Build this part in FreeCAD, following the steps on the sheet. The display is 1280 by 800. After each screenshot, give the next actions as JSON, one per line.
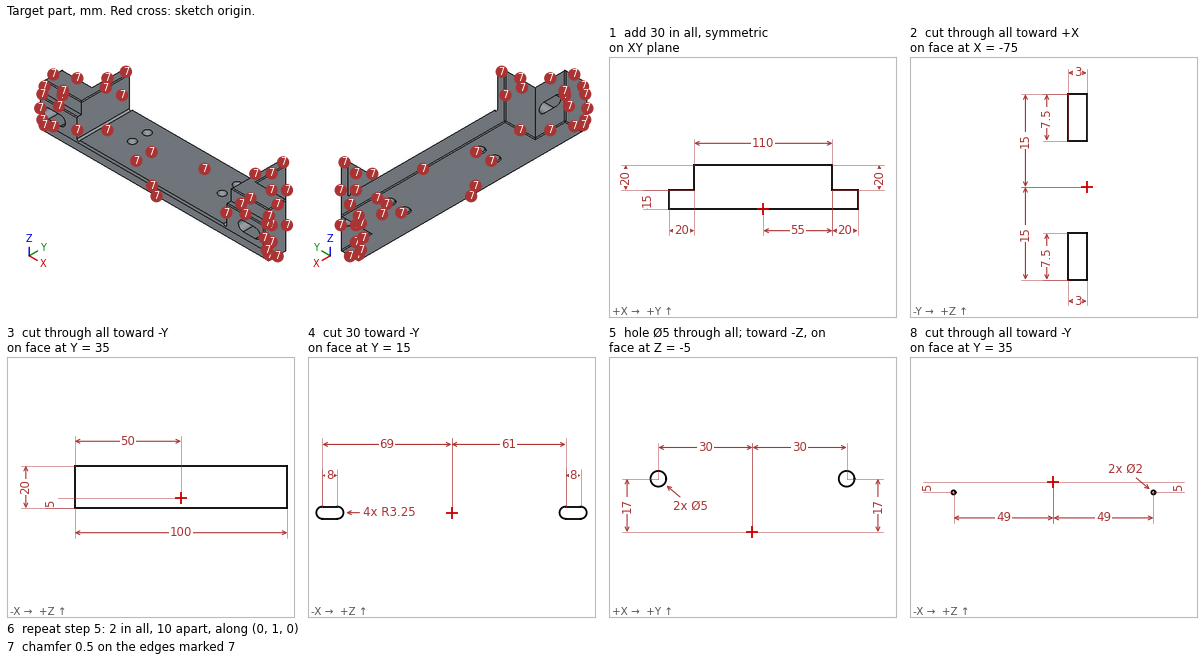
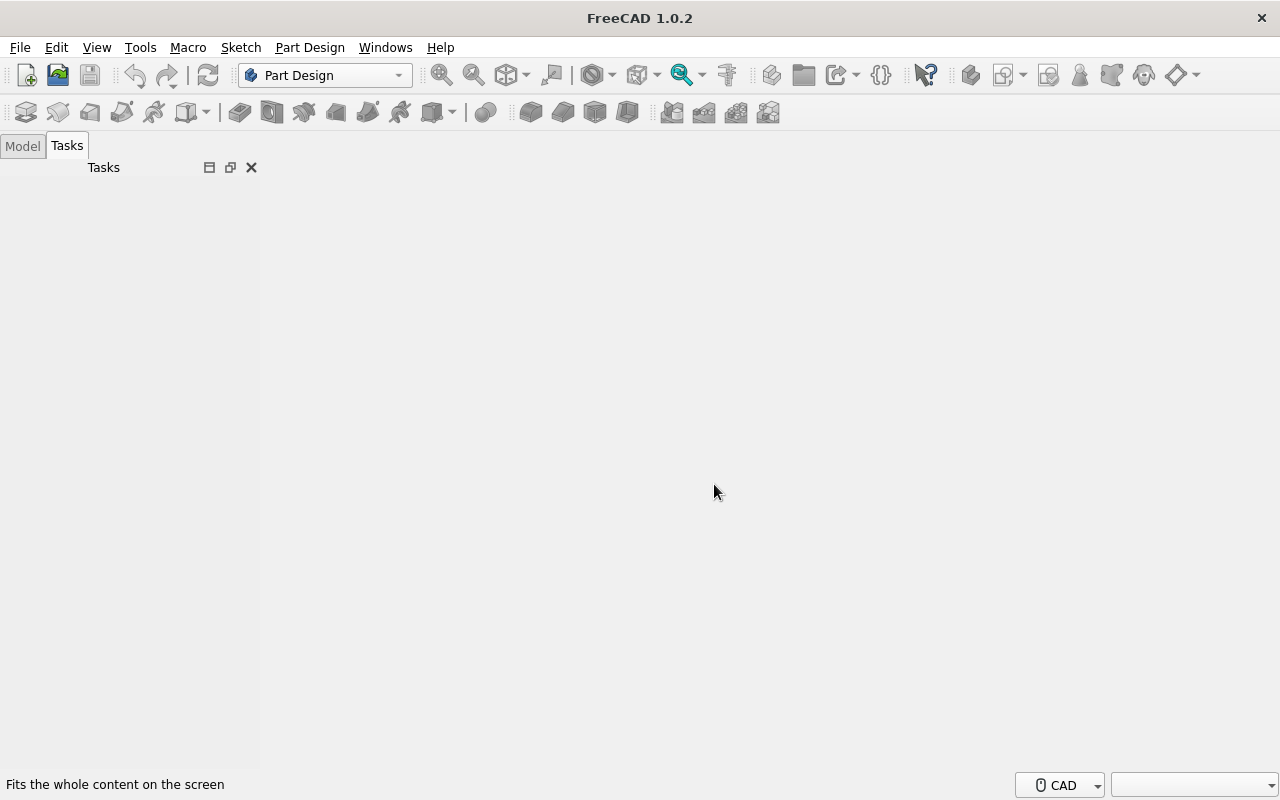
{"action": "key", "text": "ctrl+n"}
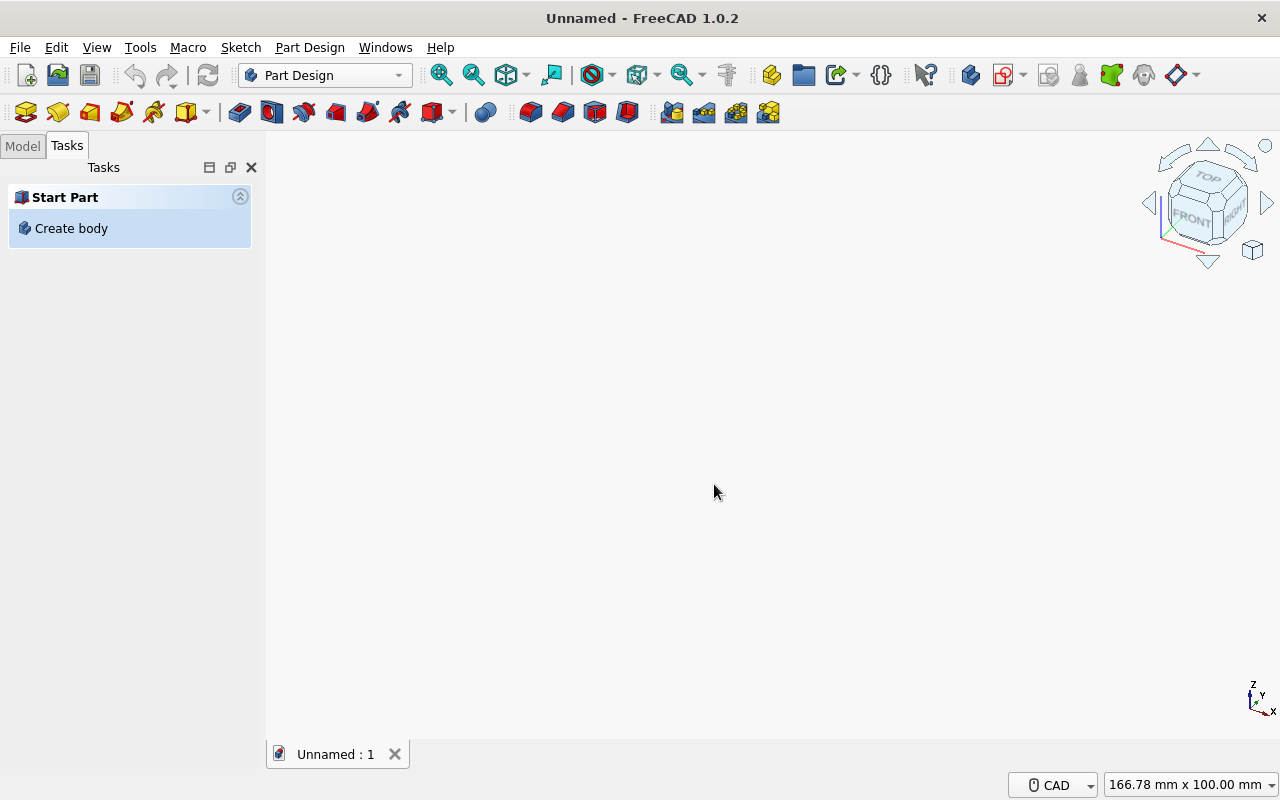
{"action": "left_click", "coordinate": [1004, 76]}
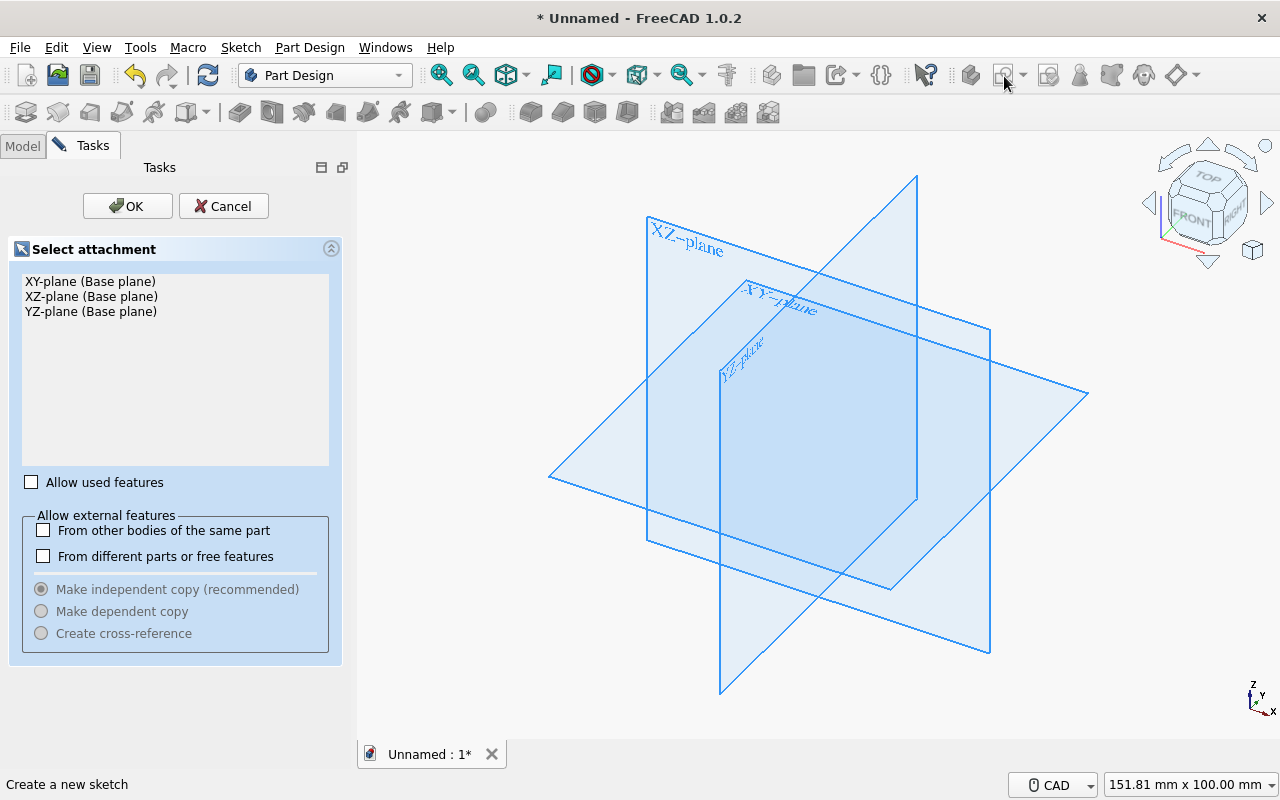
{"action": "left_click", "coordinate": [82, 282]}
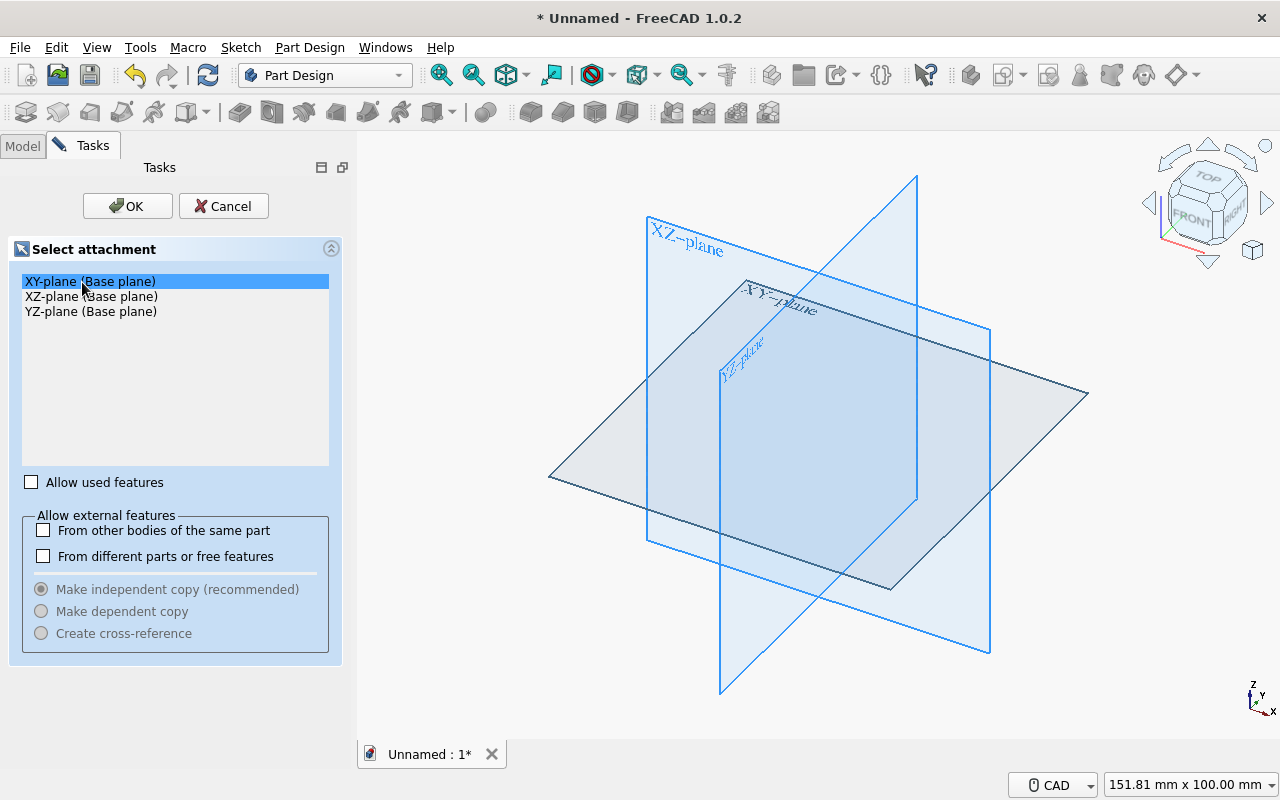
{"action": "left_click", "coordinate": [128, 206]}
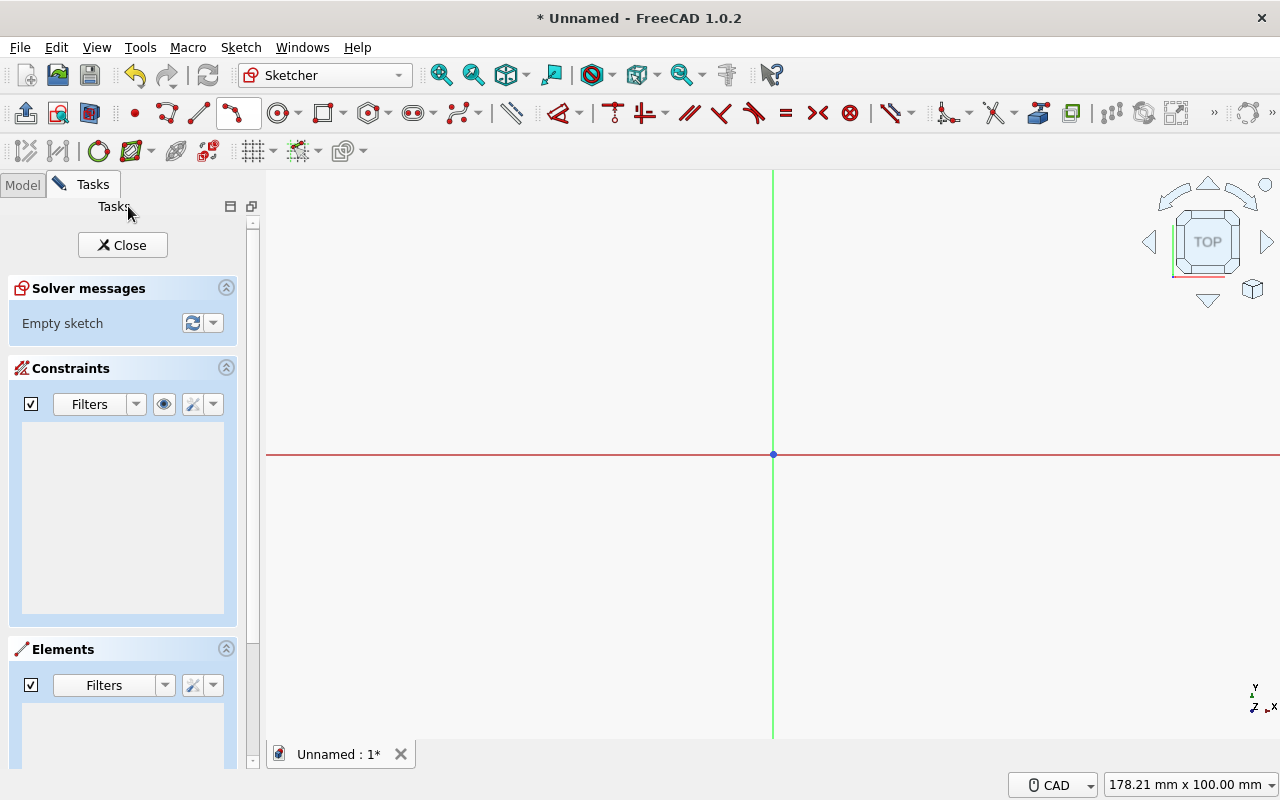
{"action": "scroll", "coordinate": [565, 657], "scroll_direction": "down", "scroll_amount": 2}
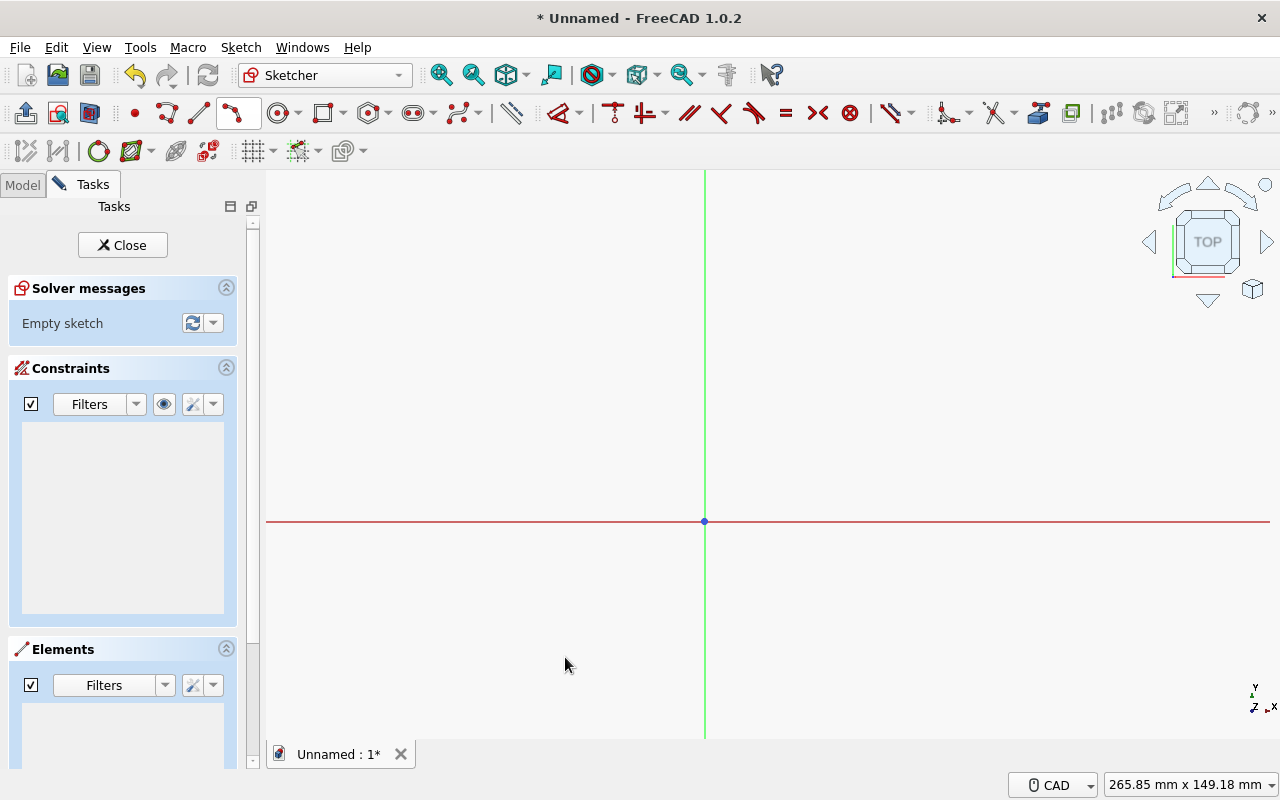
{"action": "key", "text": "g m"}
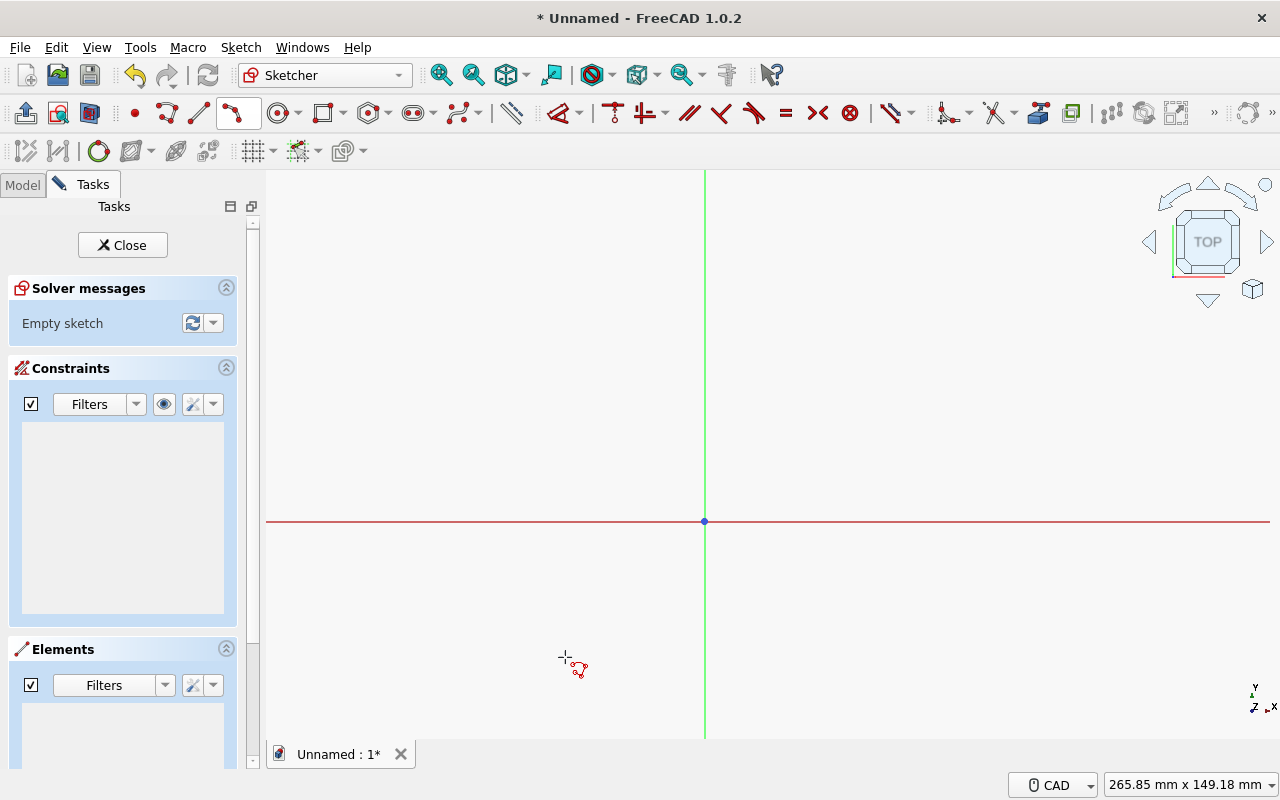
{"action": "left_click", "coordinate": [914, 464]}
{"action": "left_click", "coordinate": [914, 388]}
{"action": "left_click", "coordinate": [495, 388]}
{"action": "left_click", "coordinate": [495, 464]}
{"action": "left_click", "coordinate": [418, 464]}
{"action": "left_click", "coordinate": [418, 522]}
{"action": "left_click", "coordinate": [991, 513]}
{"action": "left_click", "coordinate": [991, 464]}
{"action": "left_click", "coordinate": [914, 465]}
{"action": "key", "text": "Escape"}
{"action": "key", "text": "Escape"}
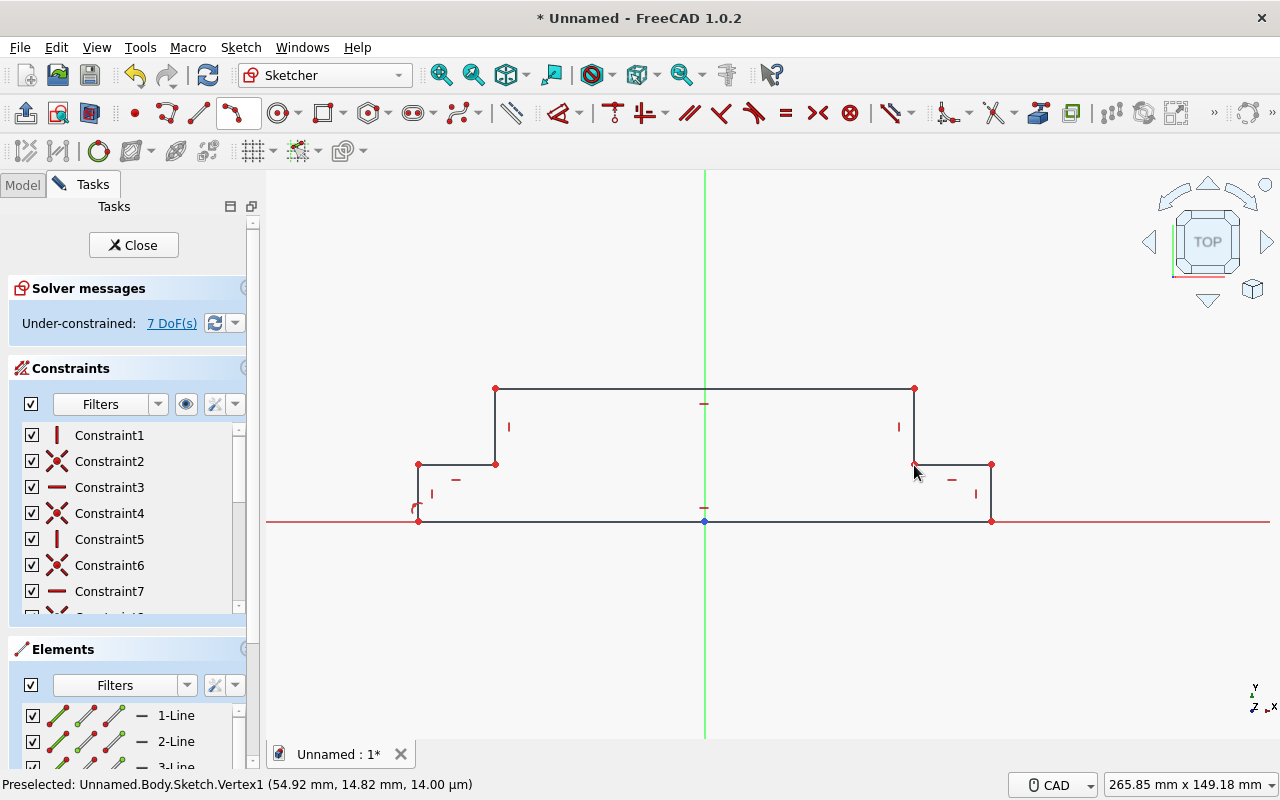
{"action": "key", "text": "d"}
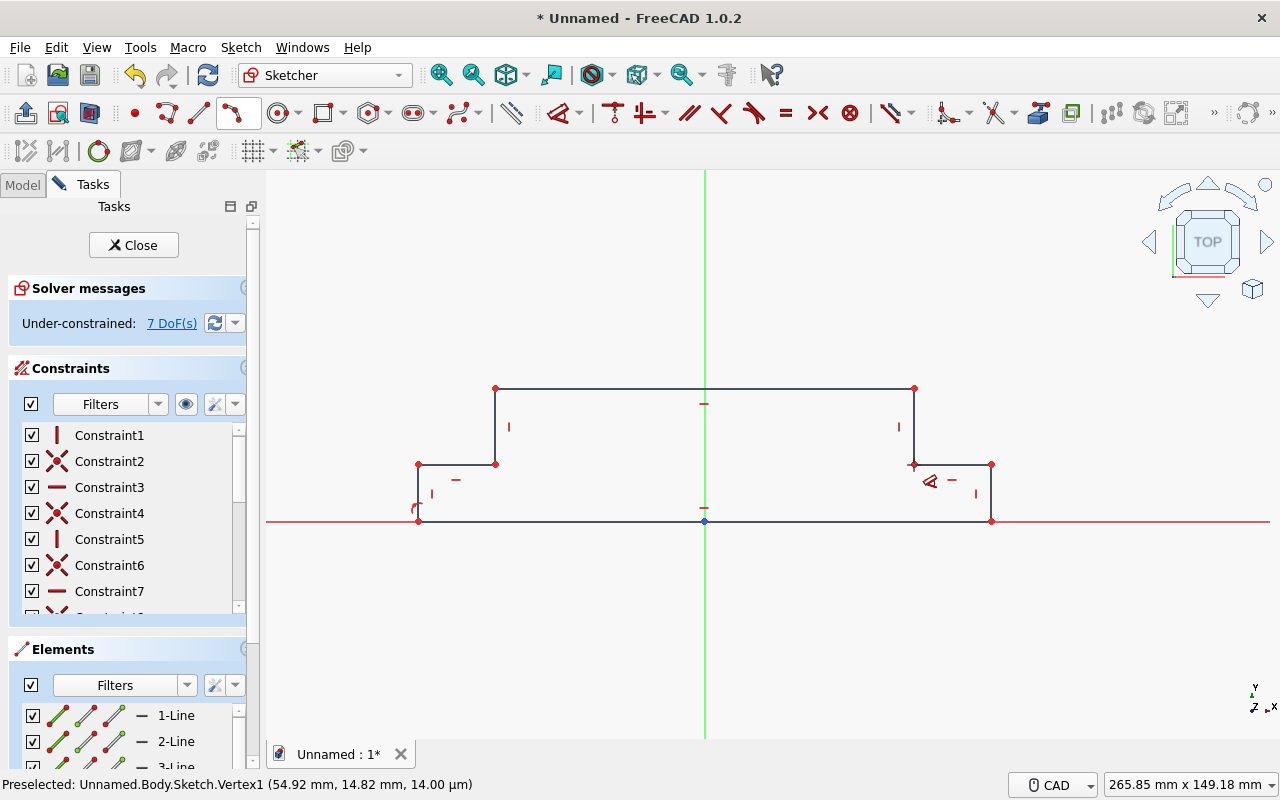
{"action": "left_click", "coordinate": [914, 442]}
{"action": "left_click", "coordinate": [948, 427]}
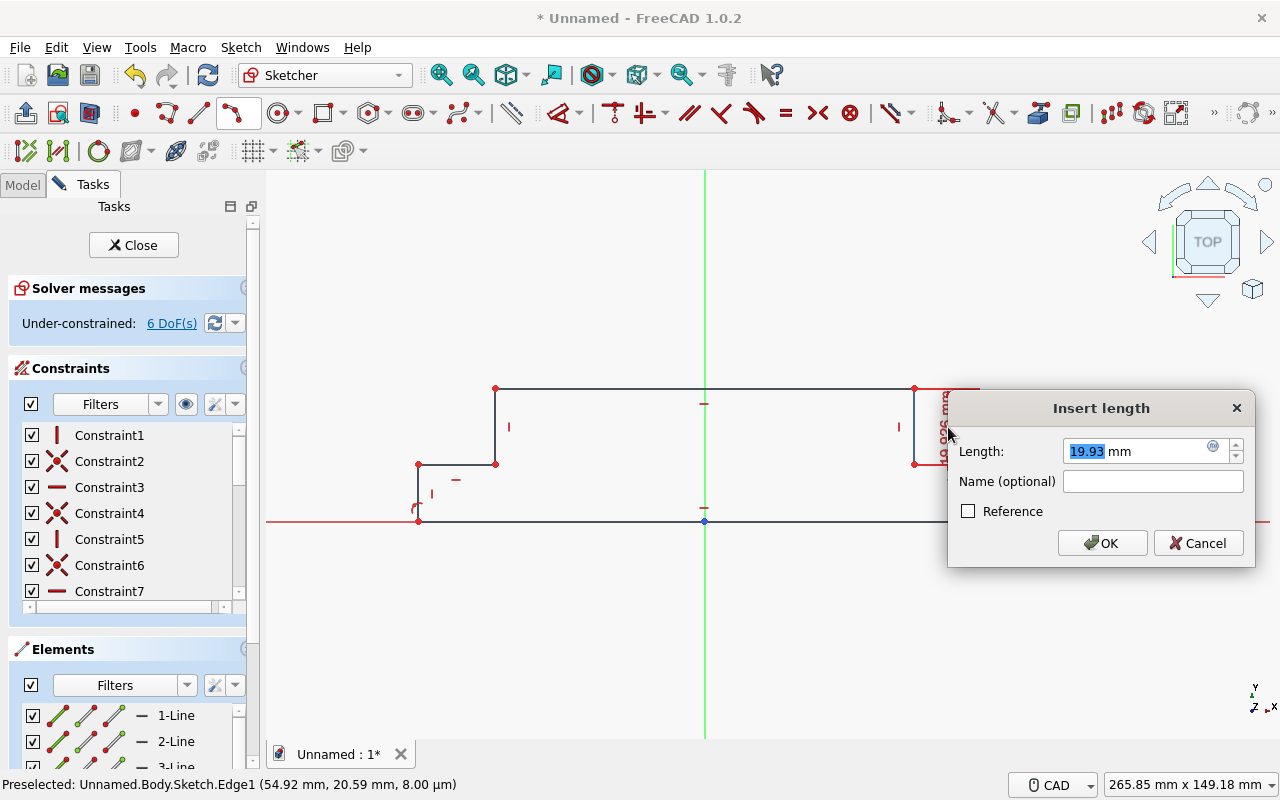
{"action": "type", "text": "20"}
{"action": "key", "text": "Return"}